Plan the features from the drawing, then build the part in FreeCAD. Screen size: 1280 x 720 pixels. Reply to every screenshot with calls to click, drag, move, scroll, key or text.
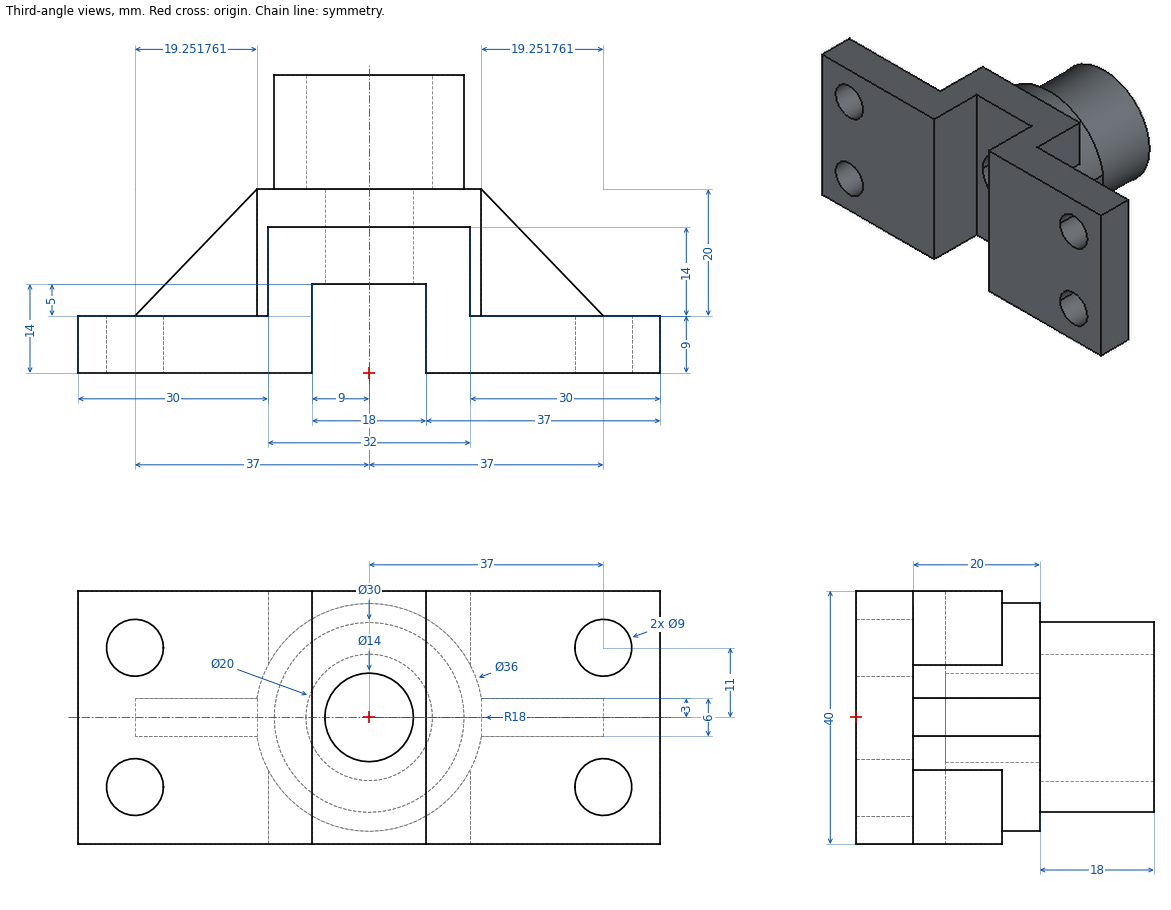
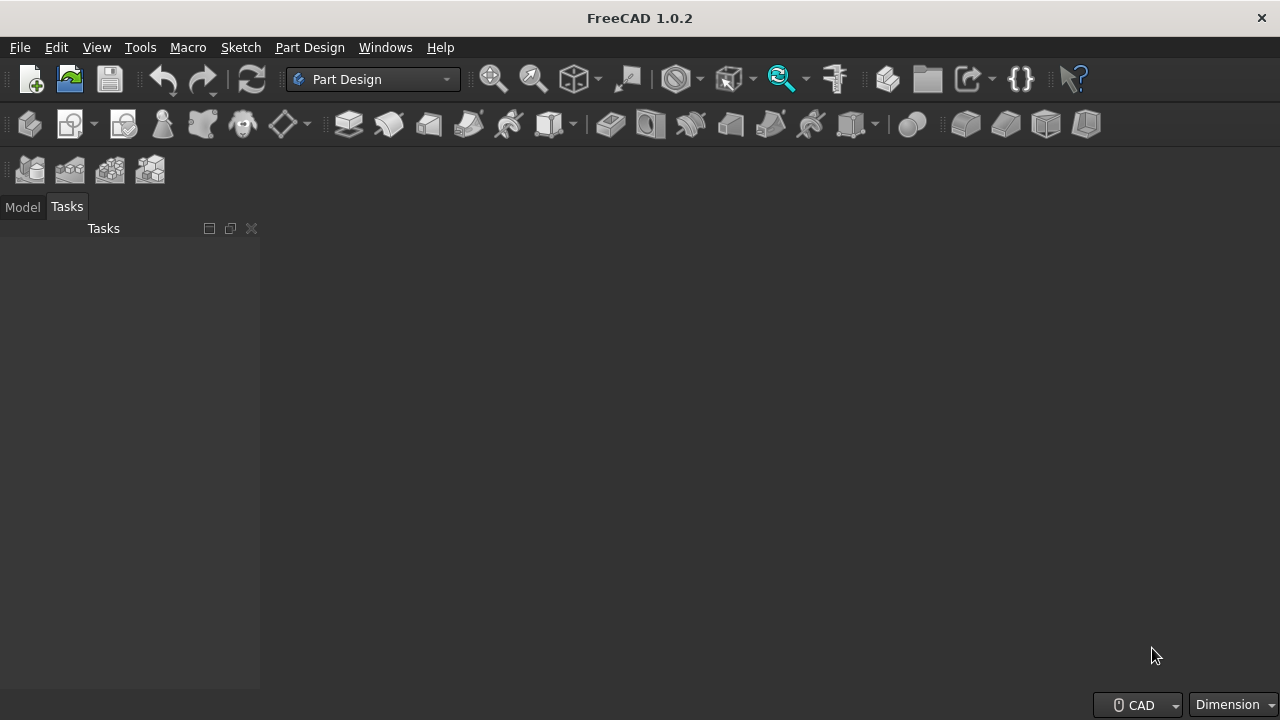
click(30, 80)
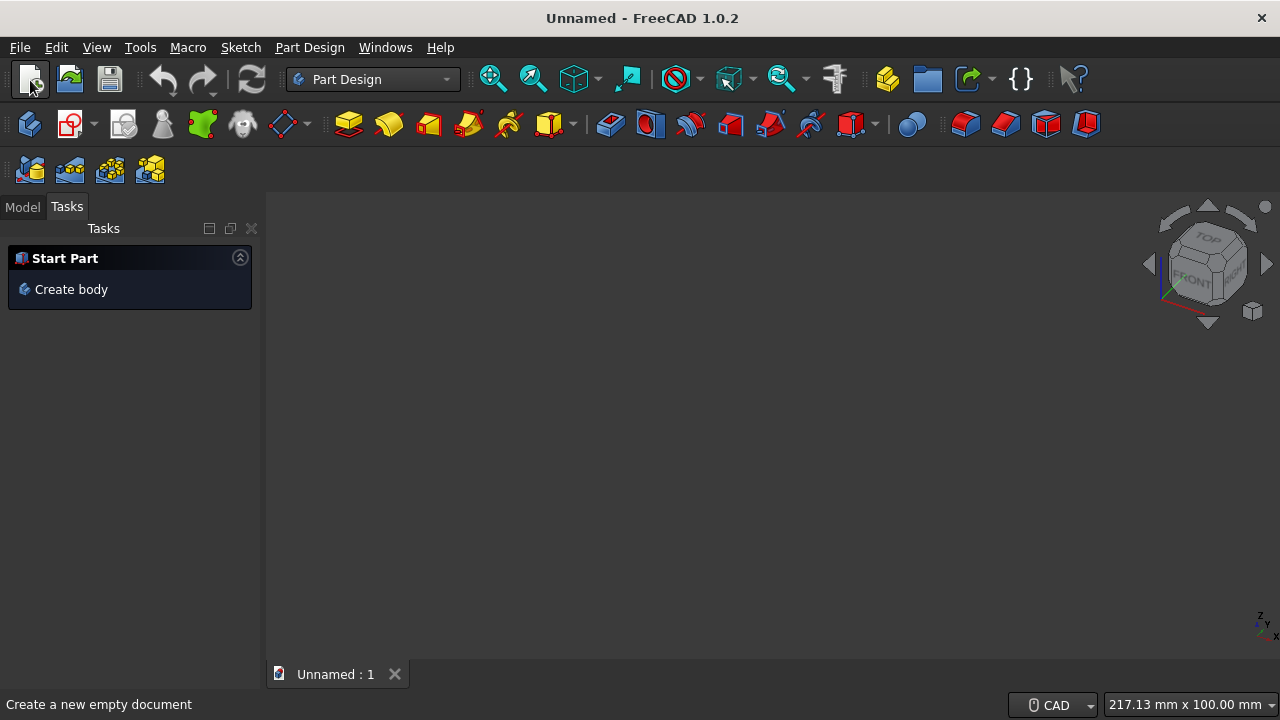
click(70, 124)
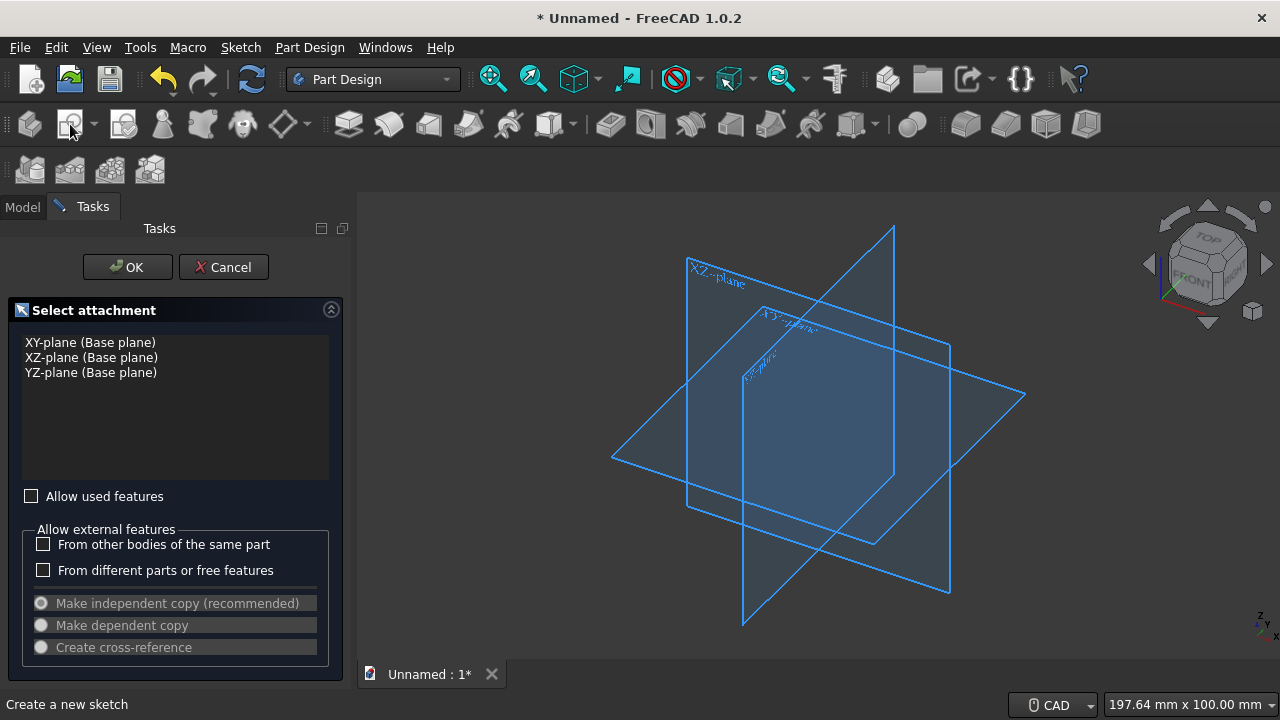
click(82, 342)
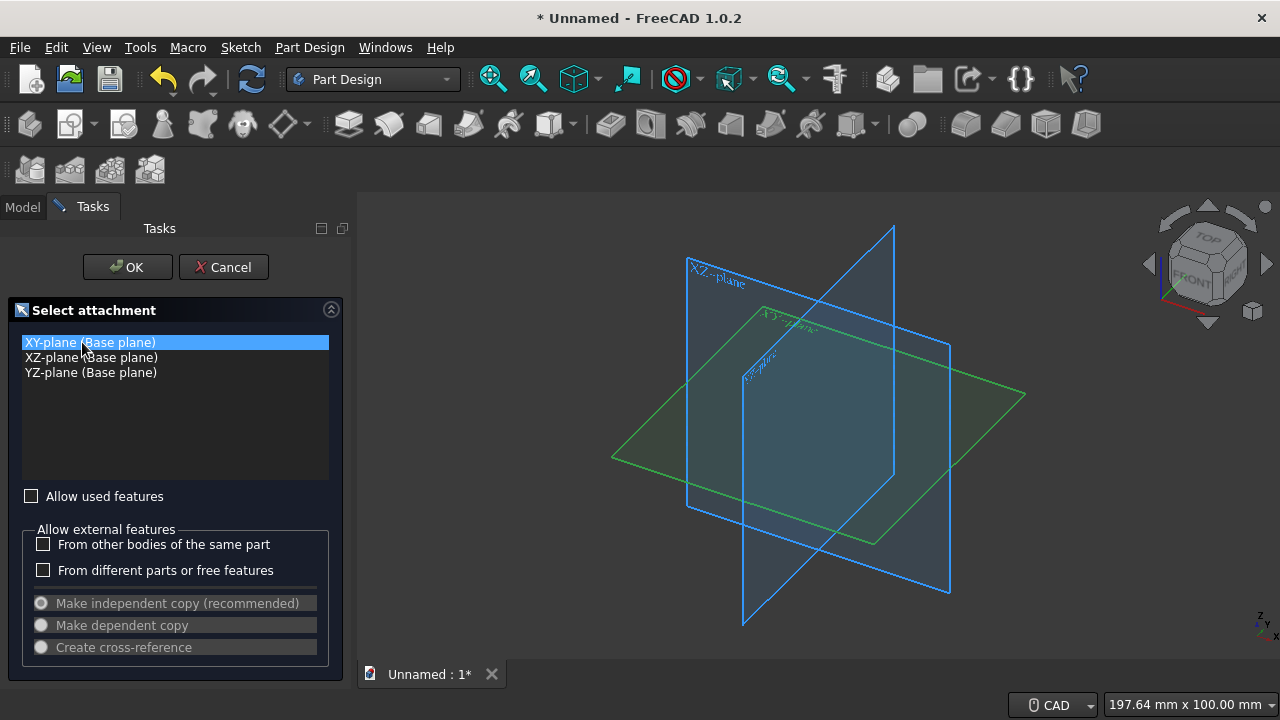
click(128, 267)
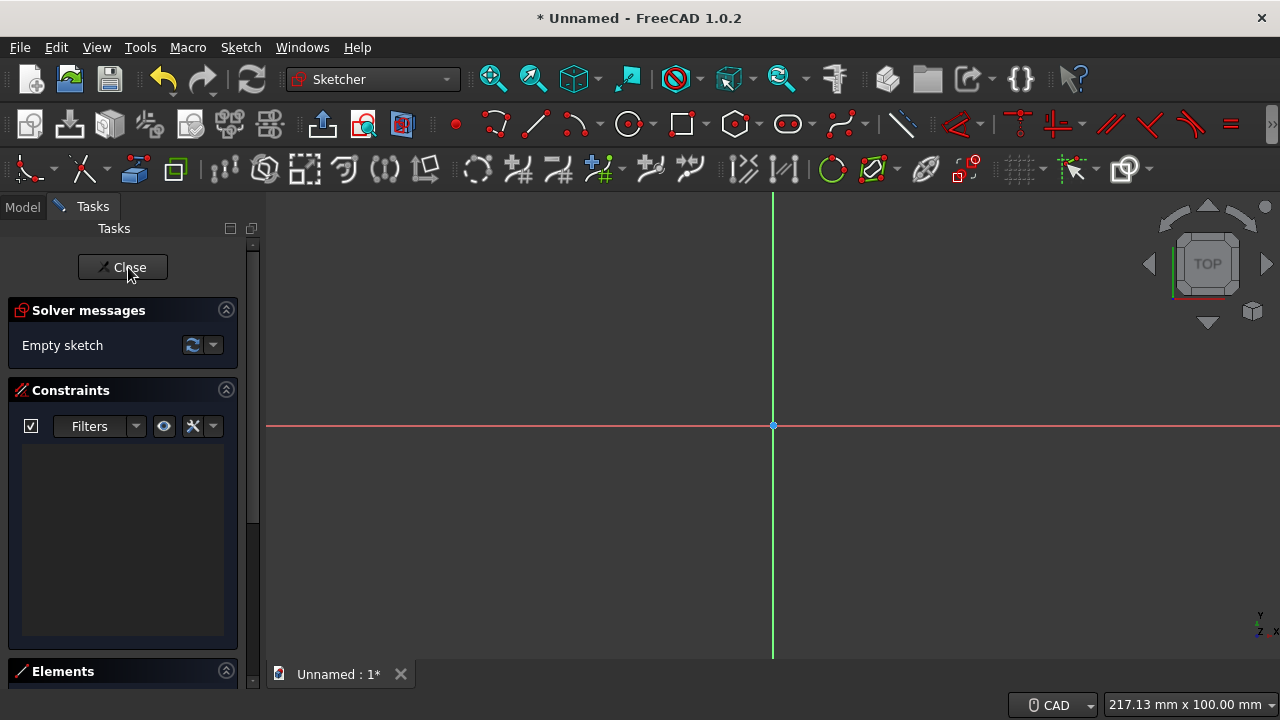
key(g)
key(m)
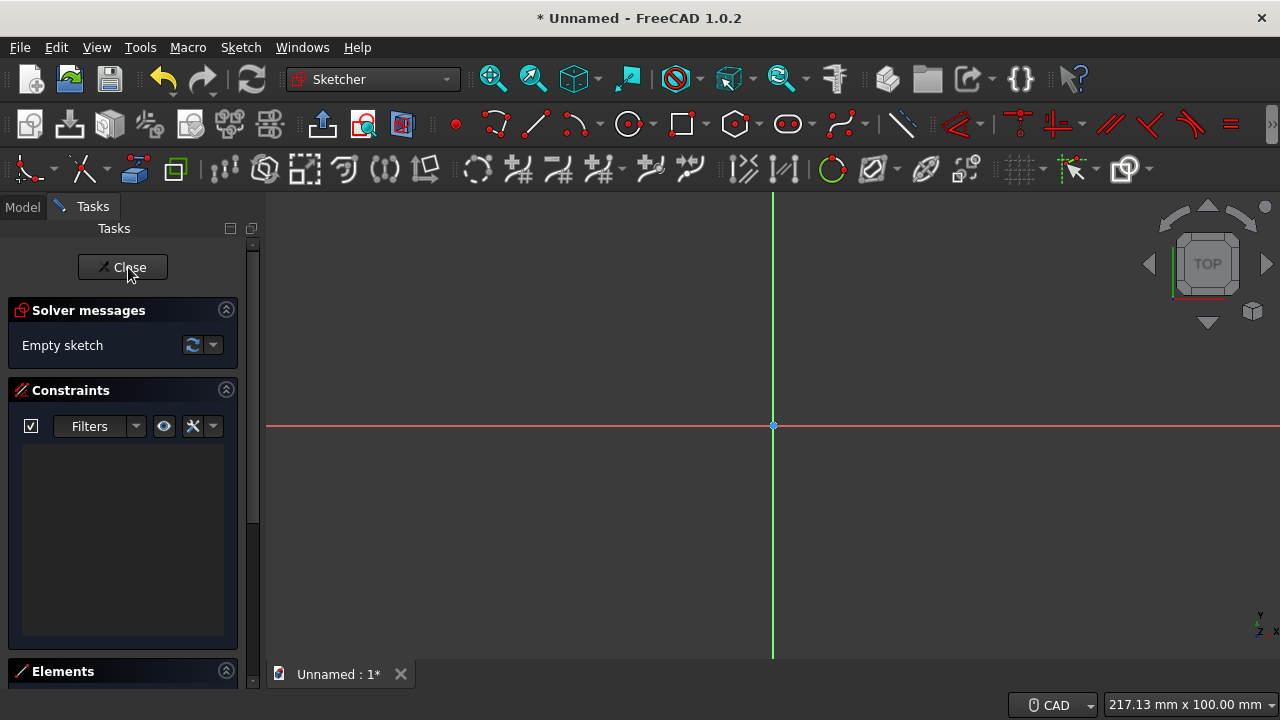
click(731, 426)
click(731, 360)
click(815, 360)
click(815, 426)
click(988, 416)
click(988, 383)
click(848, 383)
click(848, 318)
click(698, 318)
click(698, 383)
click(558, 383)
click(558, 416)
click(731, 426)
key(Escape)
key(Escape)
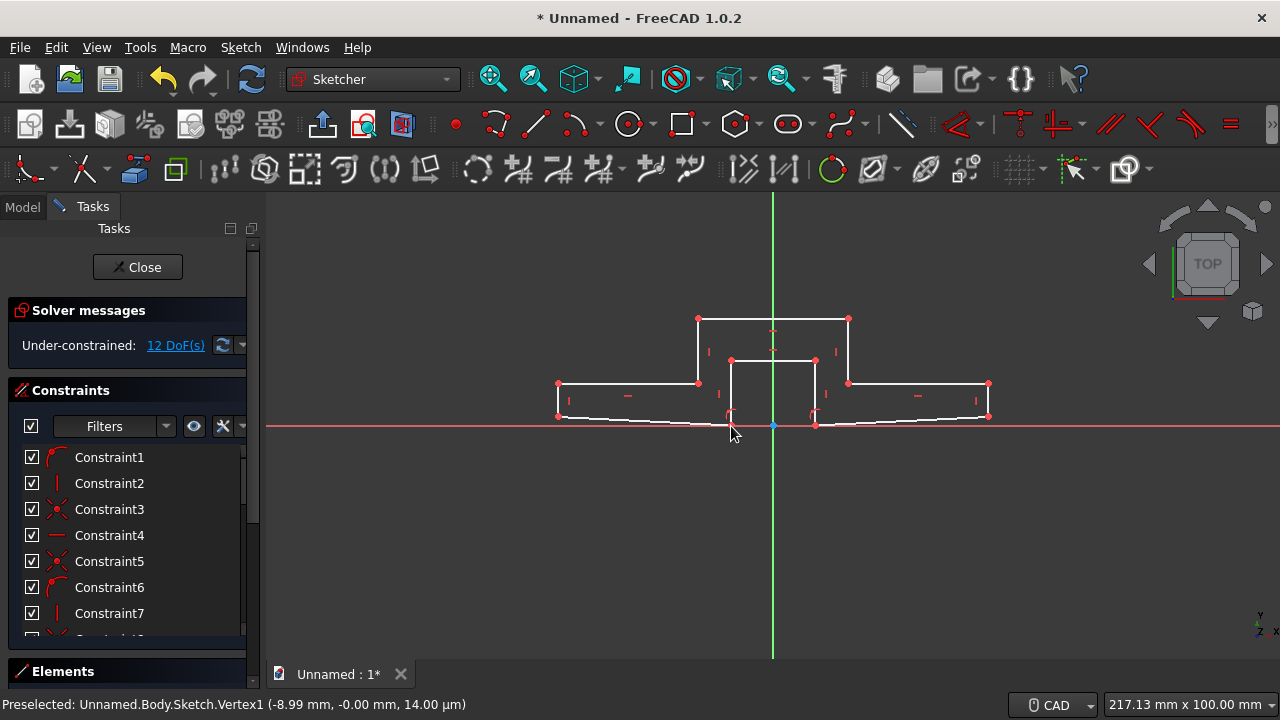
click(867, 423)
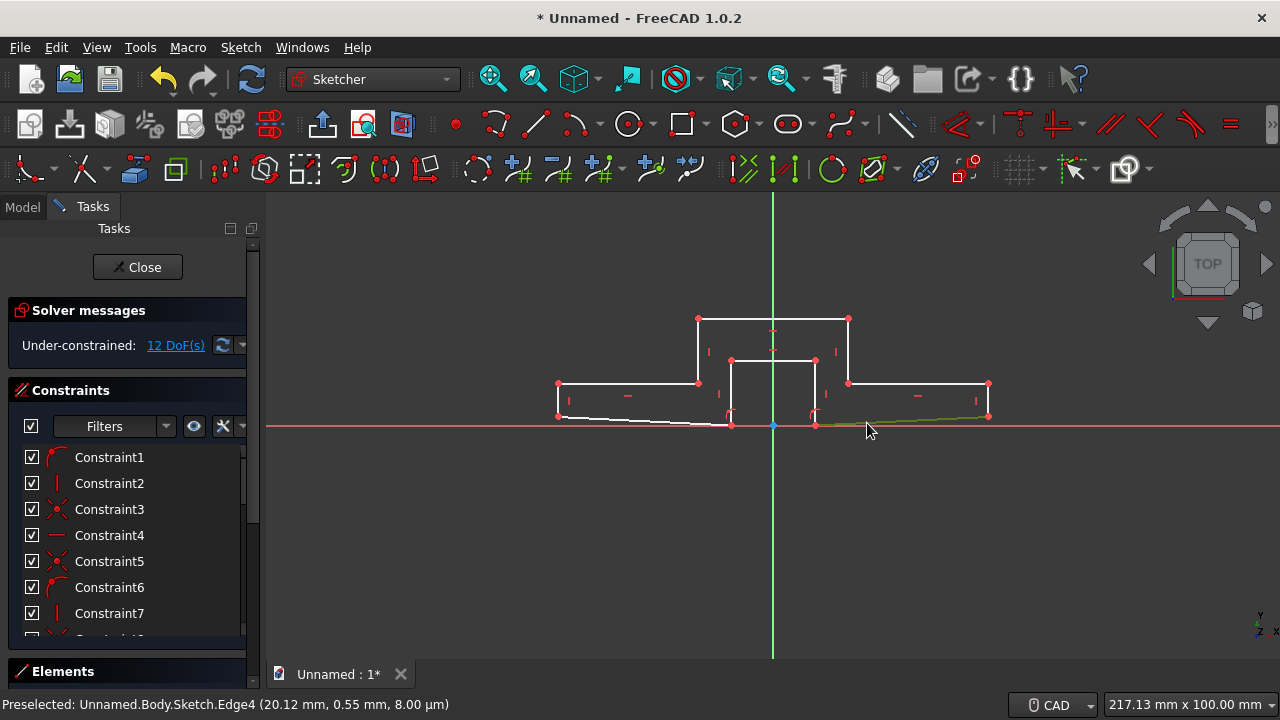
click(1084, 124)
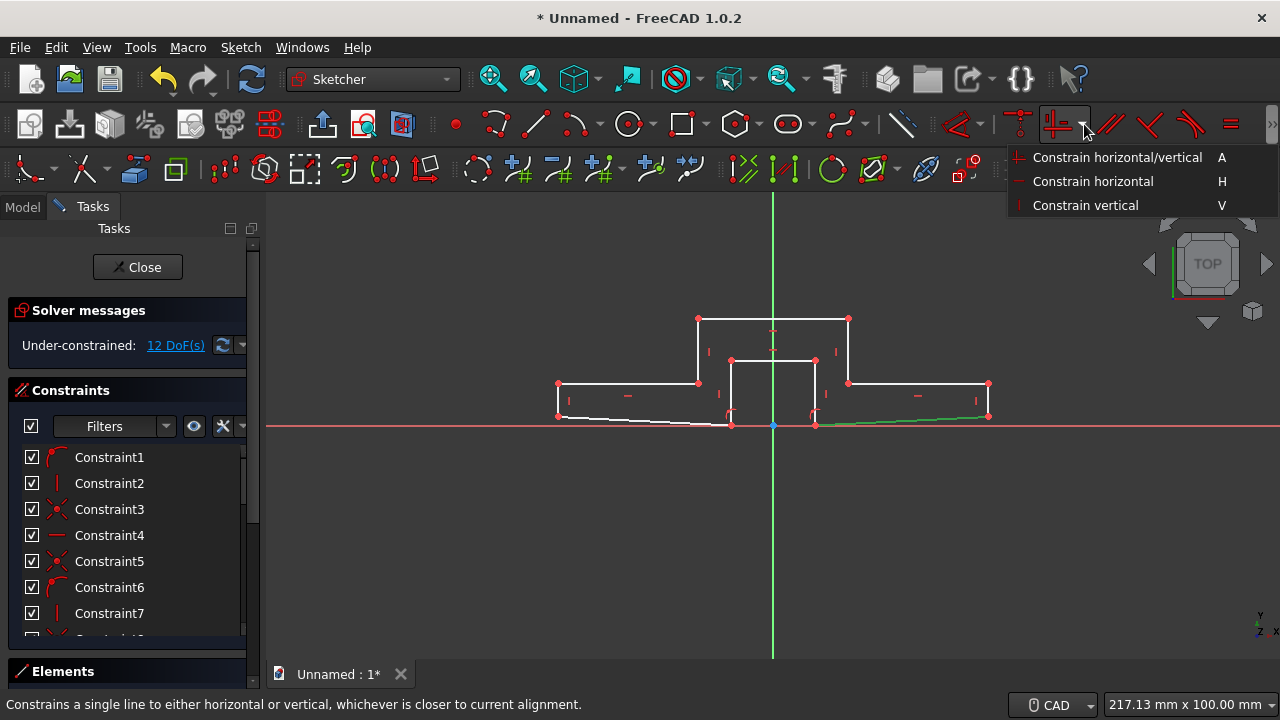
click(1143, 181)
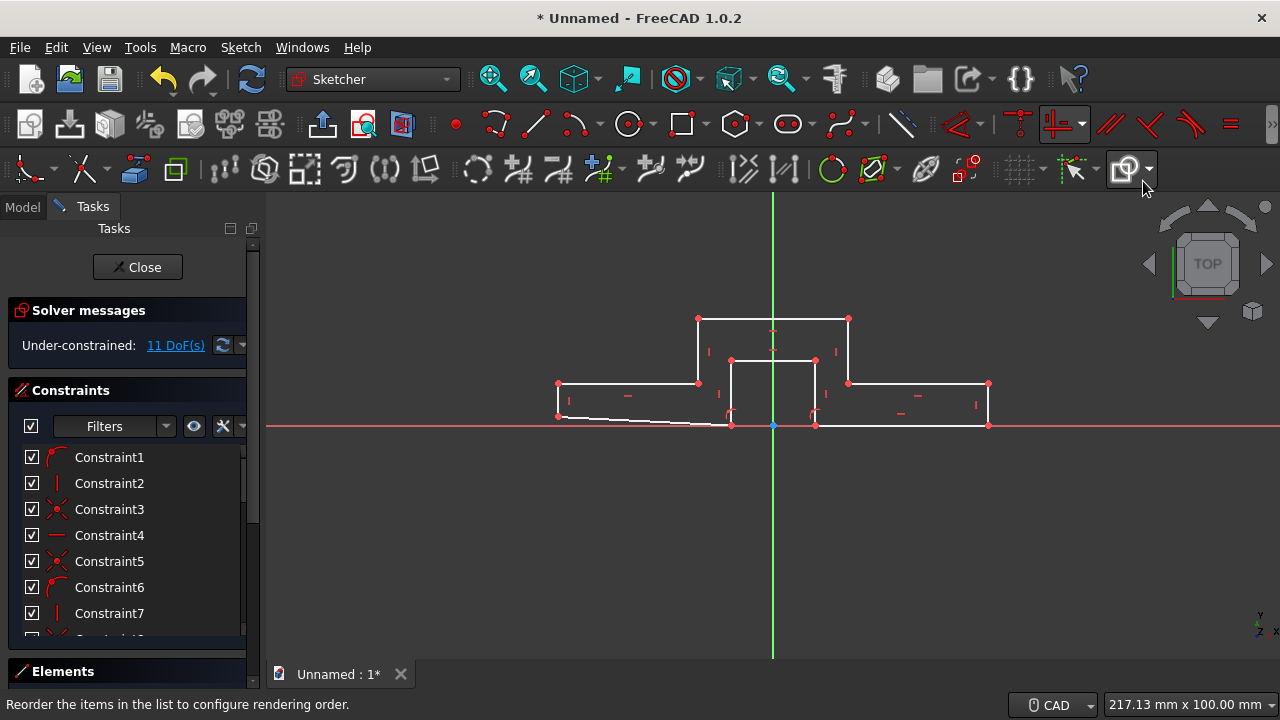
click(679, 423)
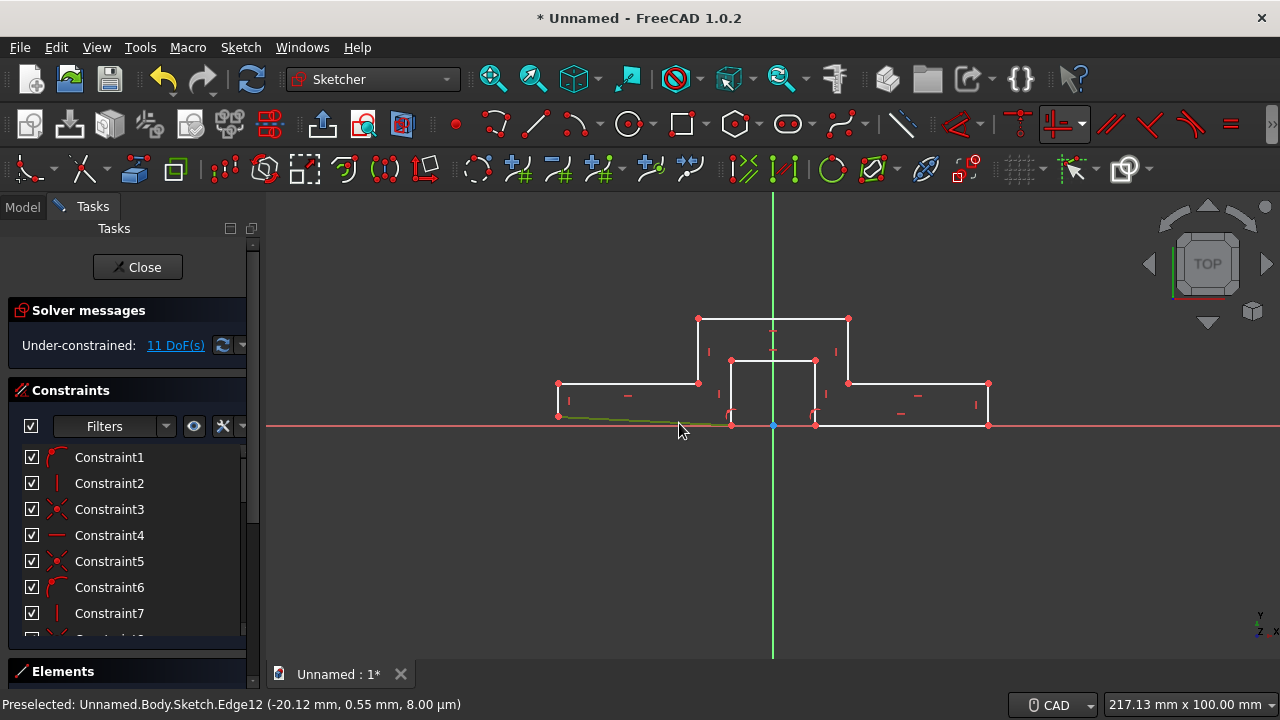
key(h)